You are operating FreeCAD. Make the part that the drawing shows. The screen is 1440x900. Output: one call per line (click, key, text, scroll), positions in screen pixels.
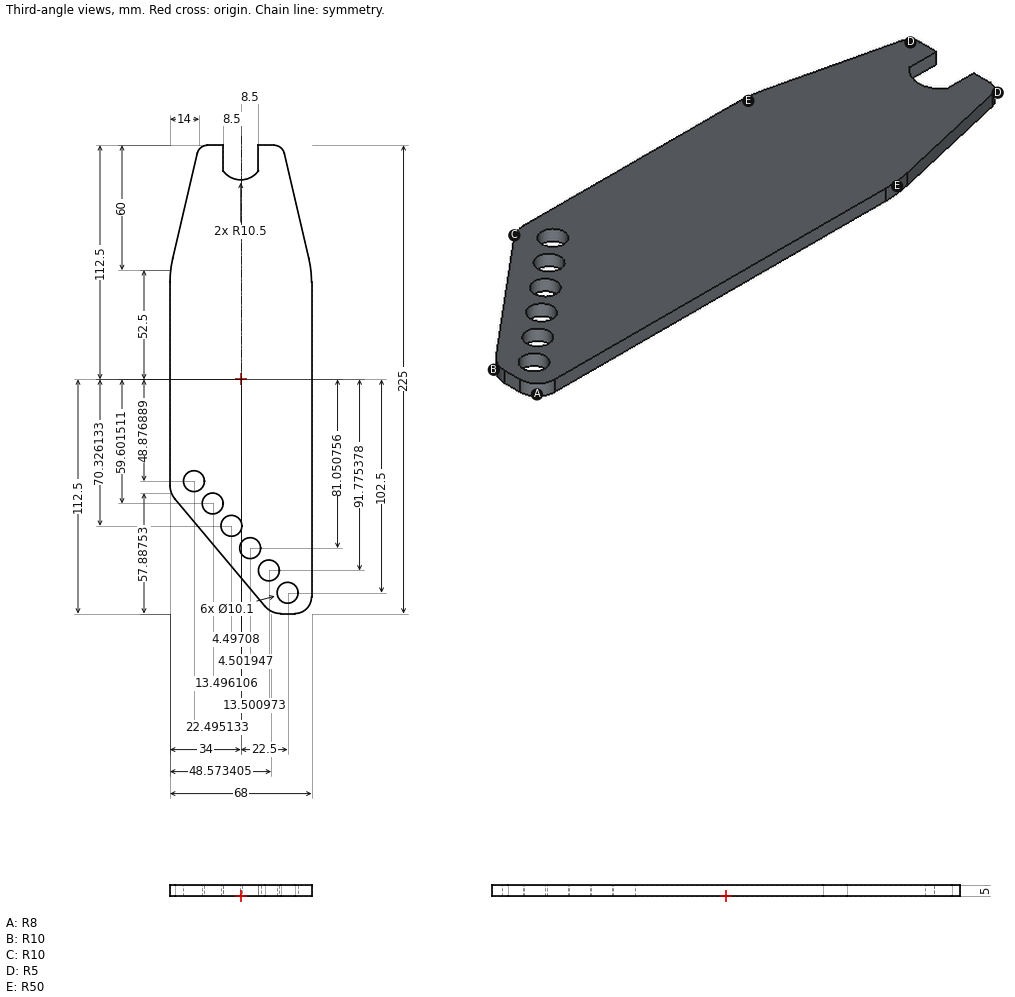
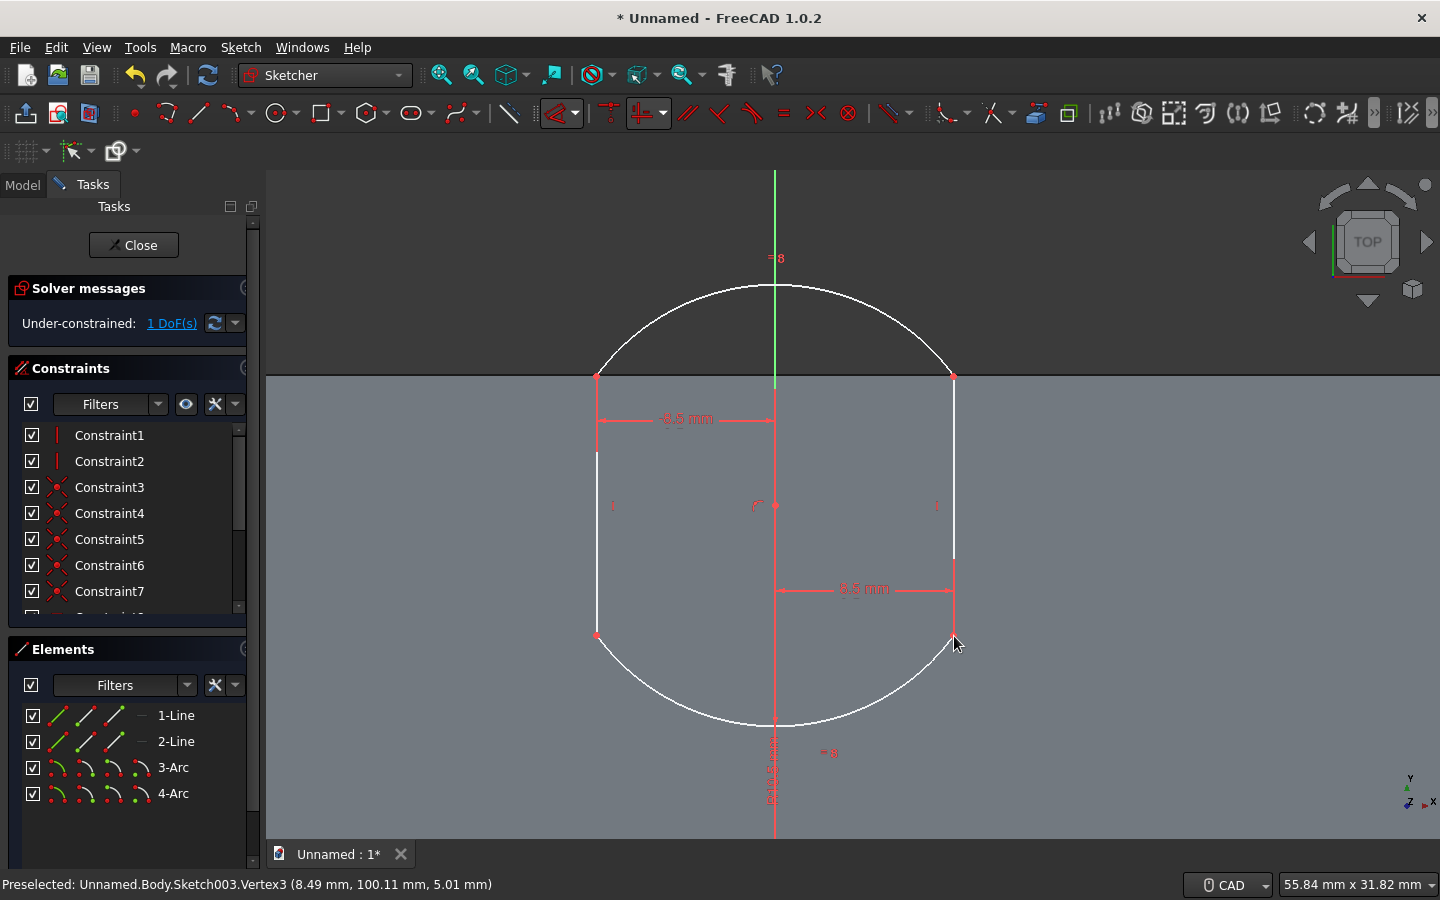
click(597, 376)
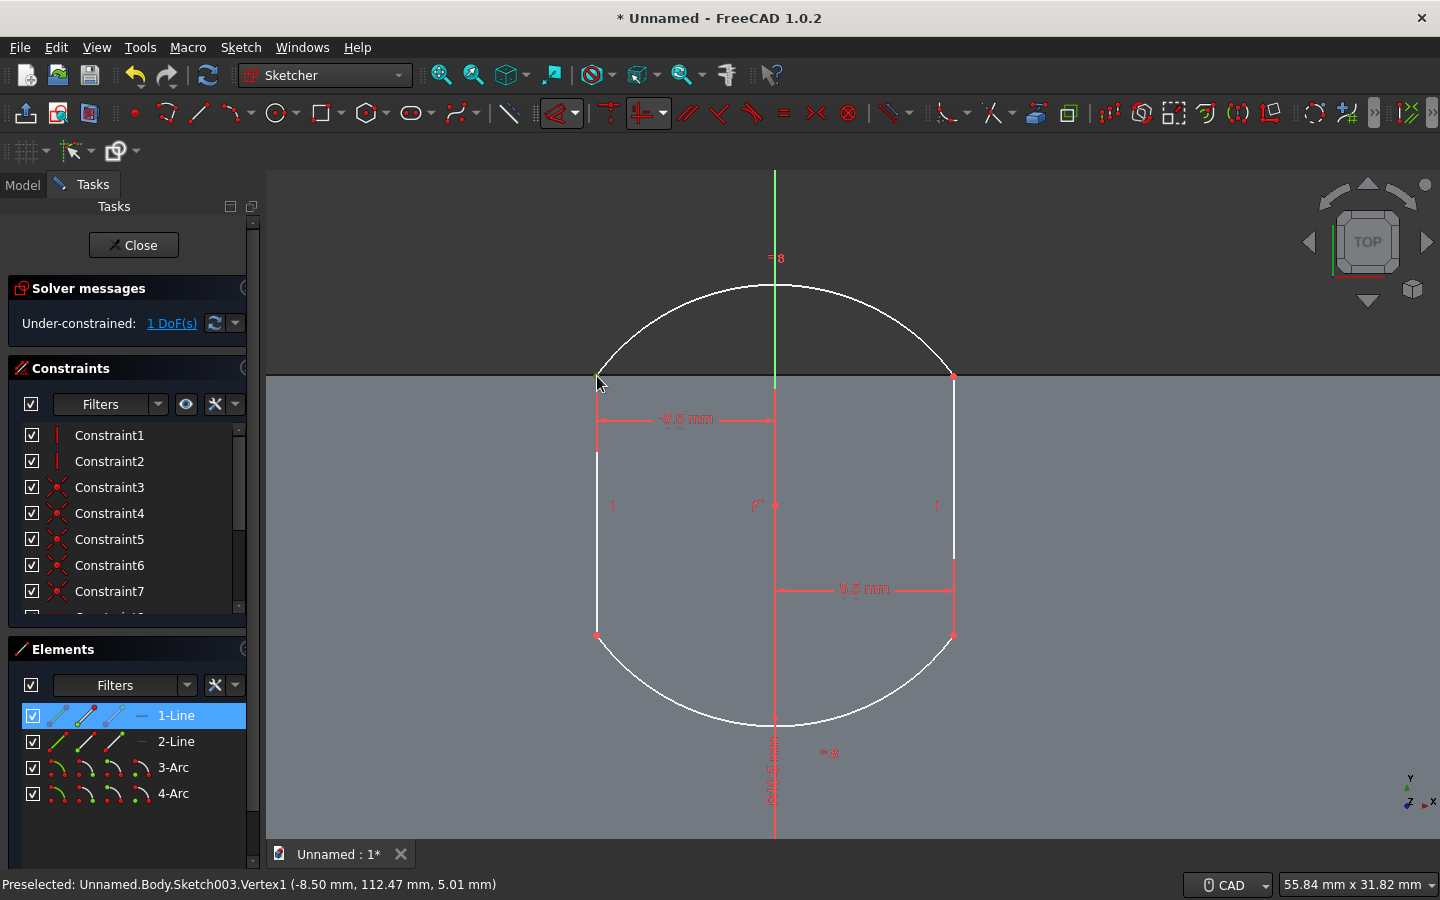
key(i)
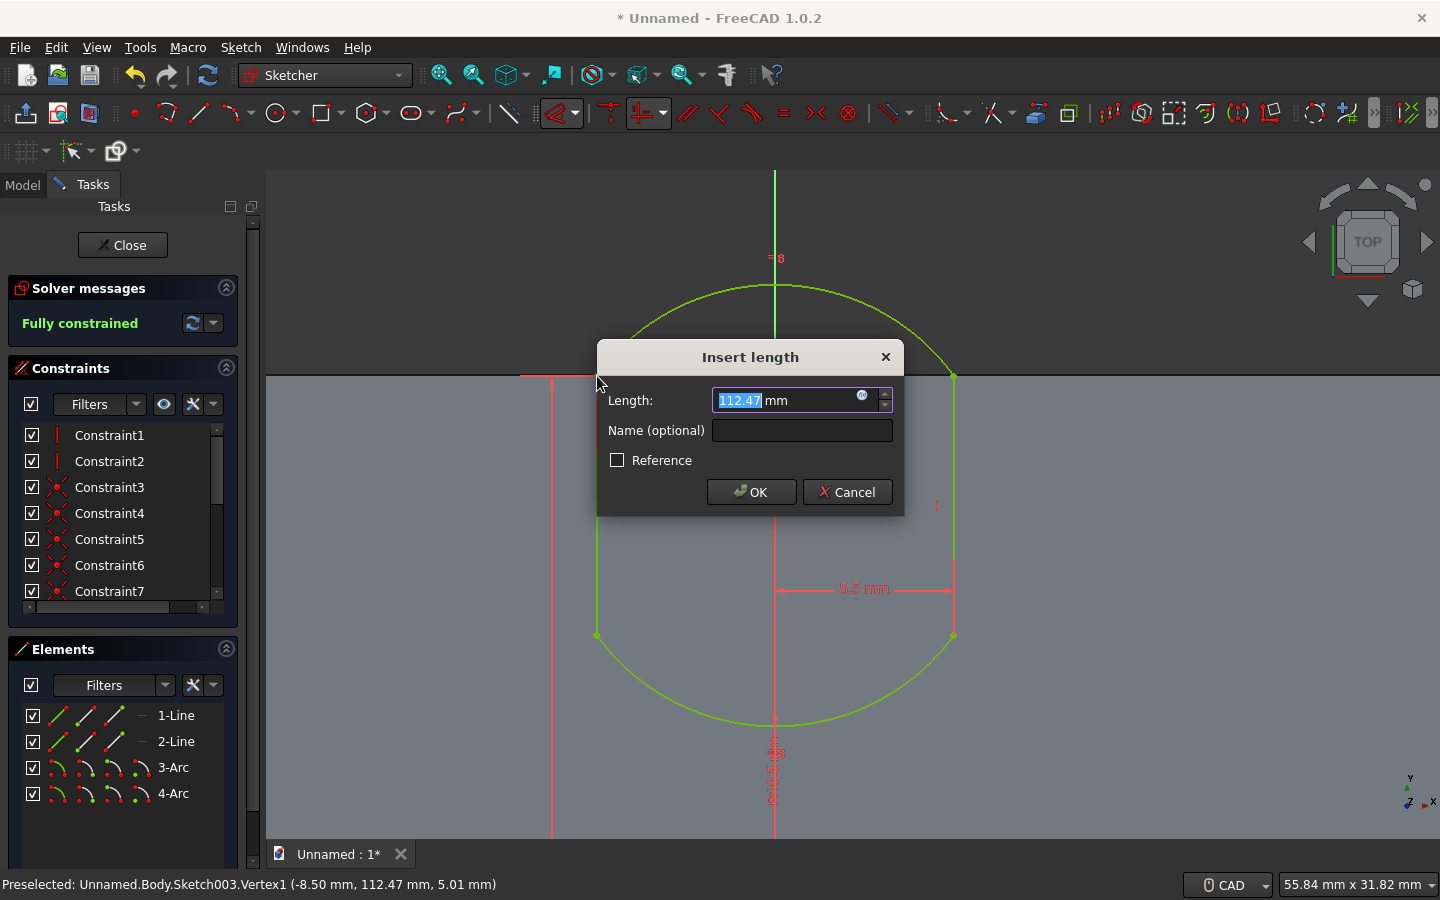
text(112.5)
key(Return)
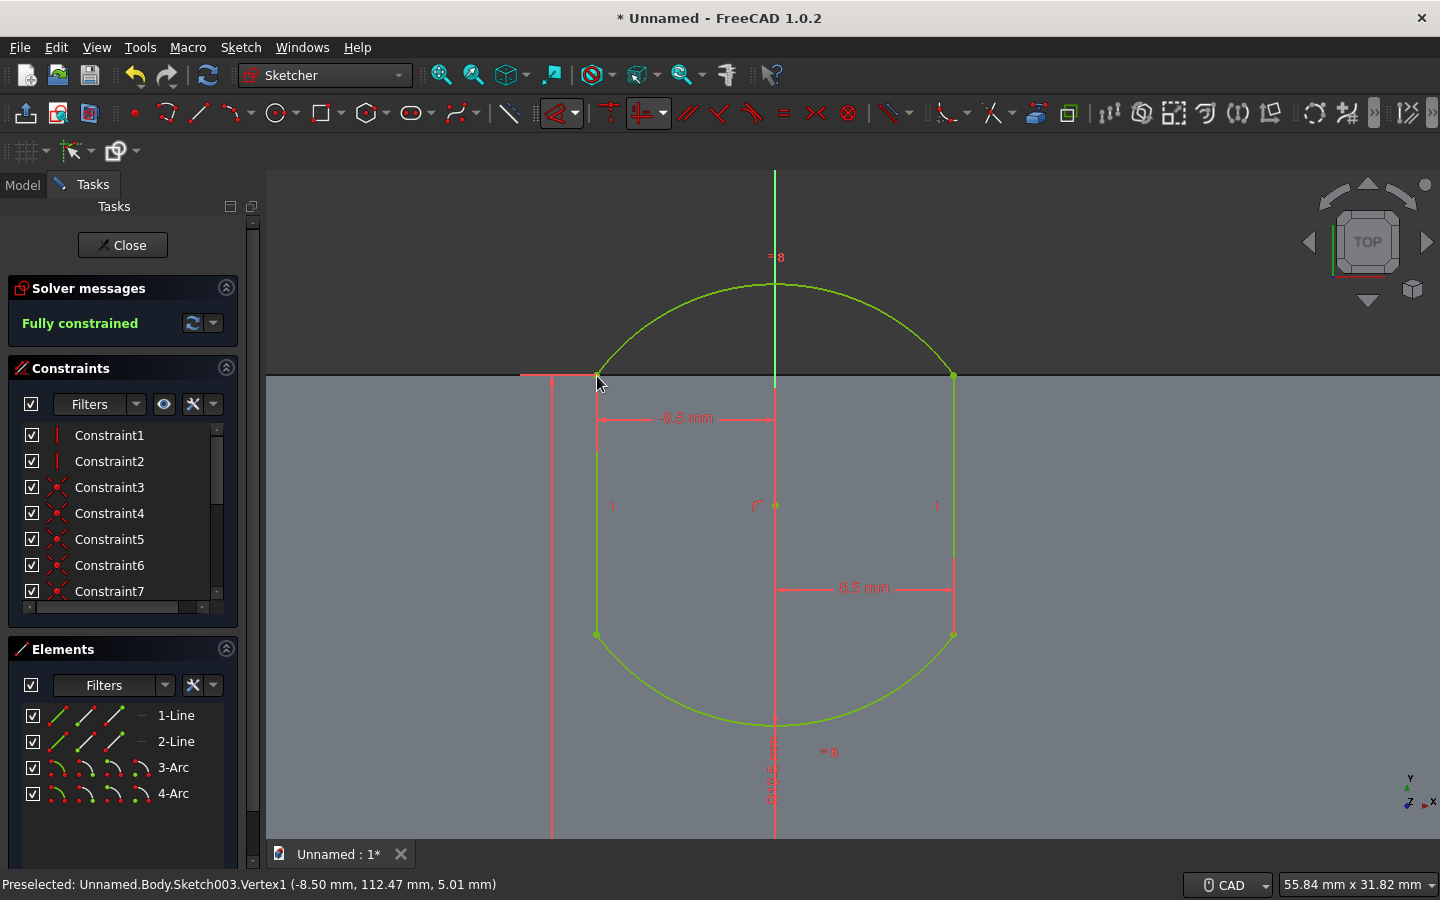
click(123, 245)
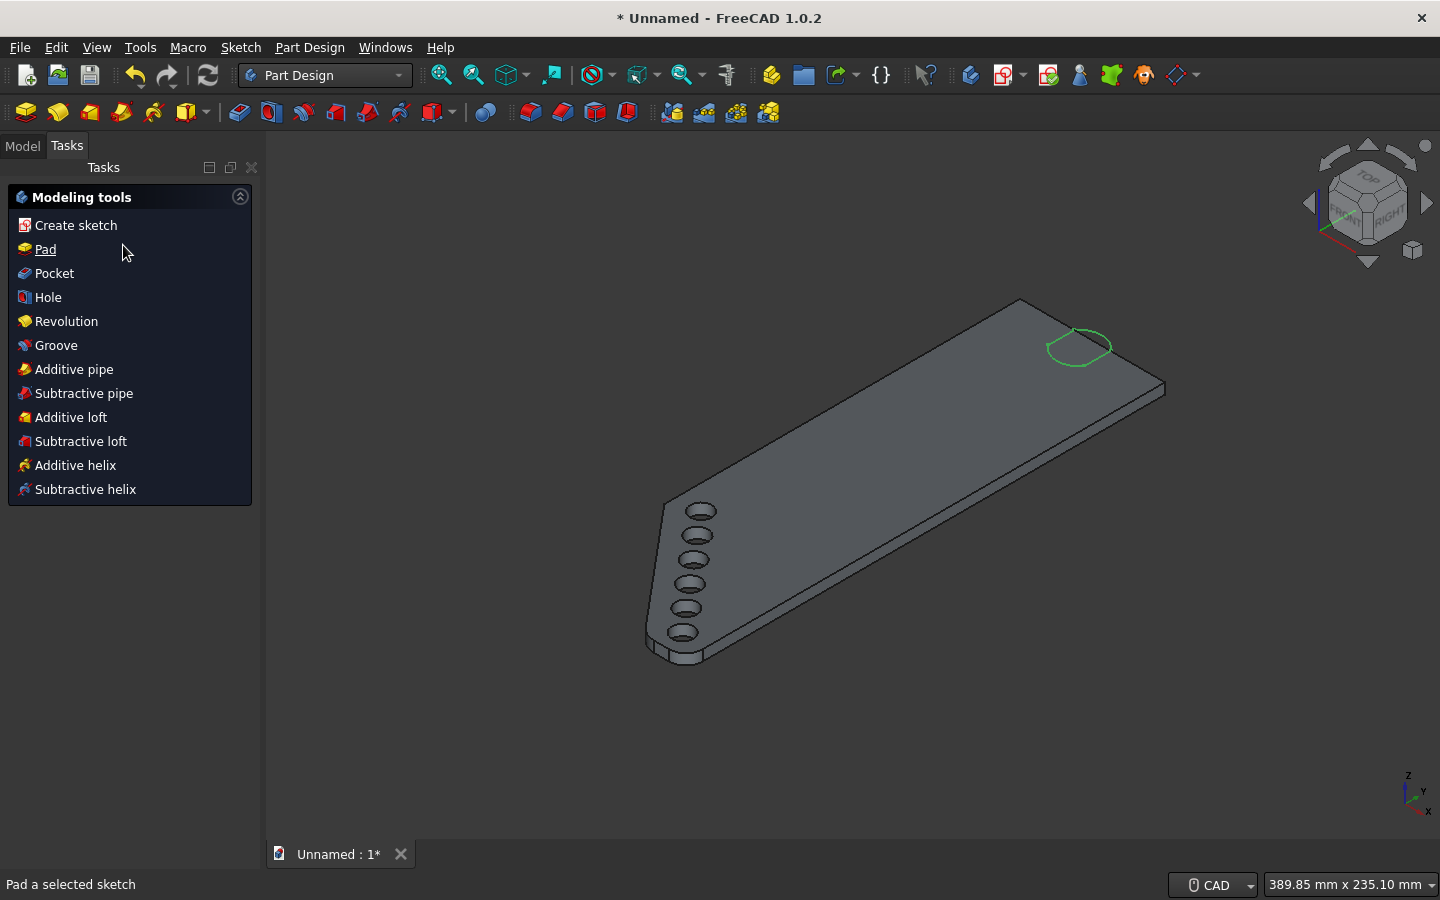
click(240, 112)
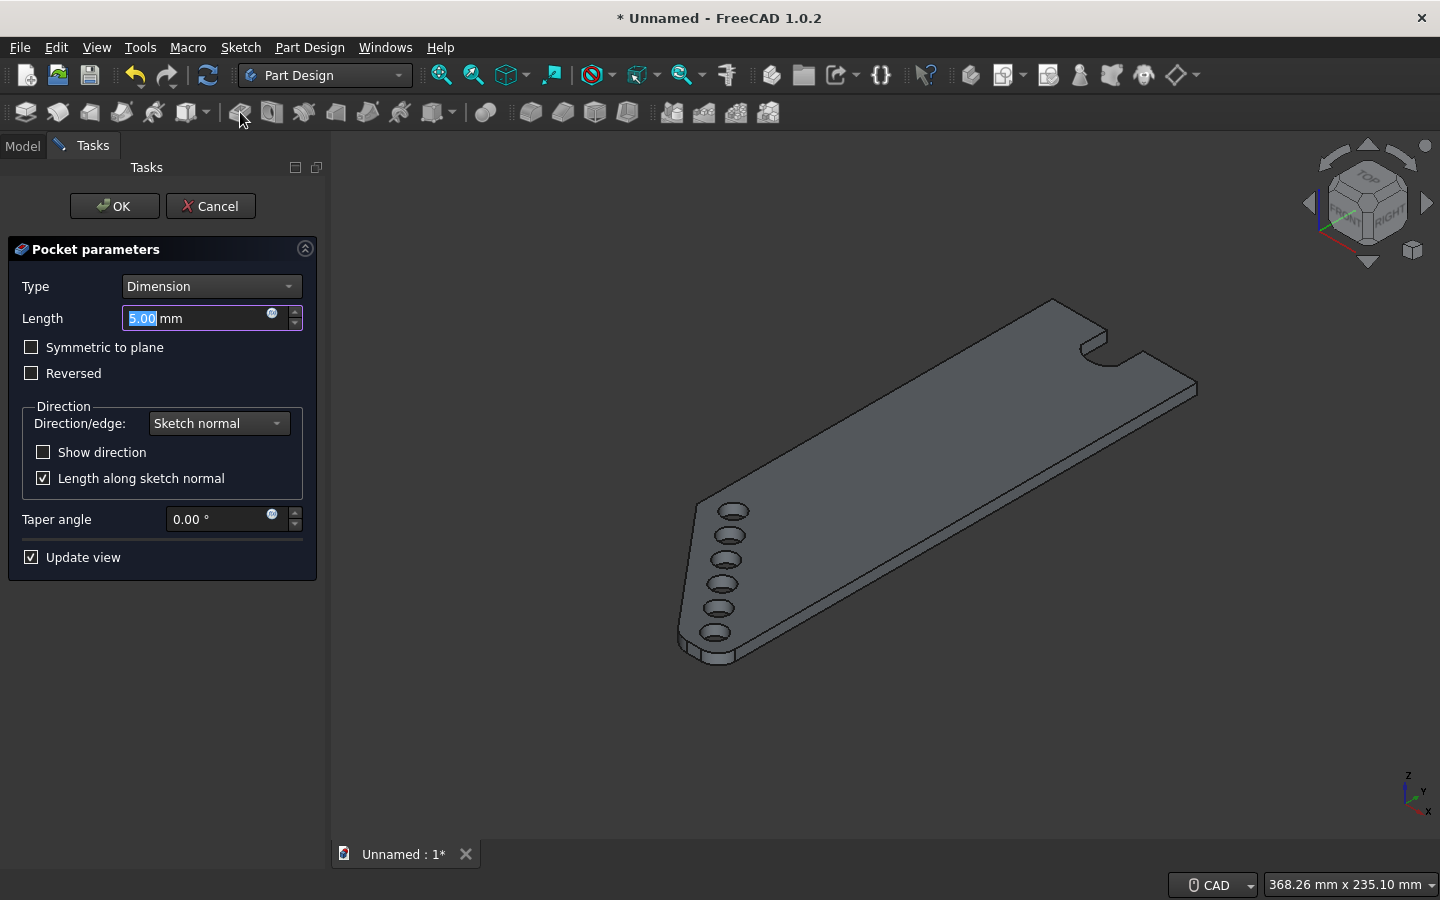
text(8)
key(Tab)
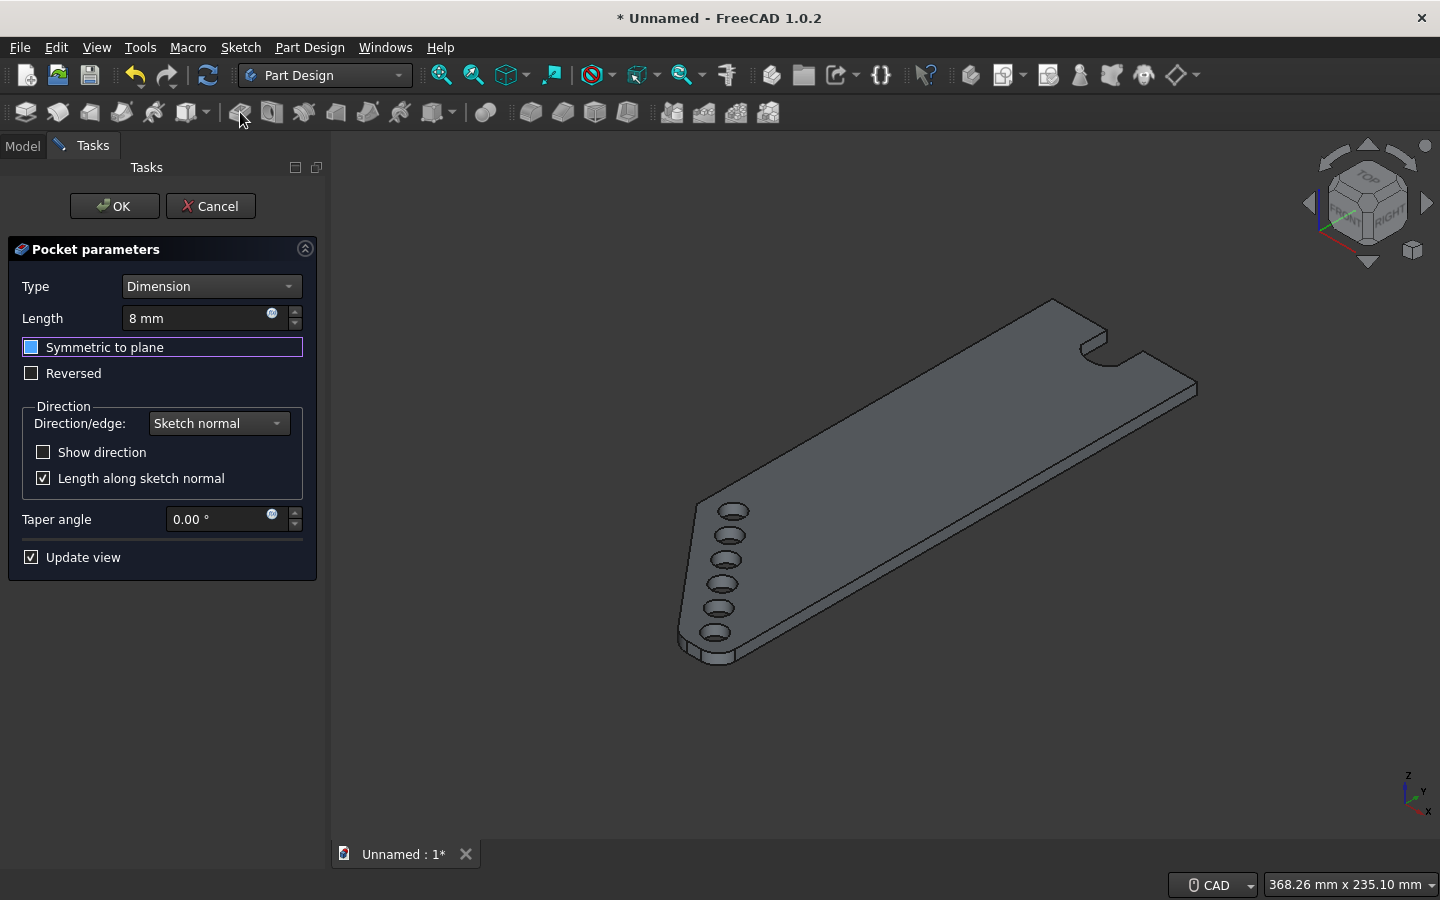
click(115, 206)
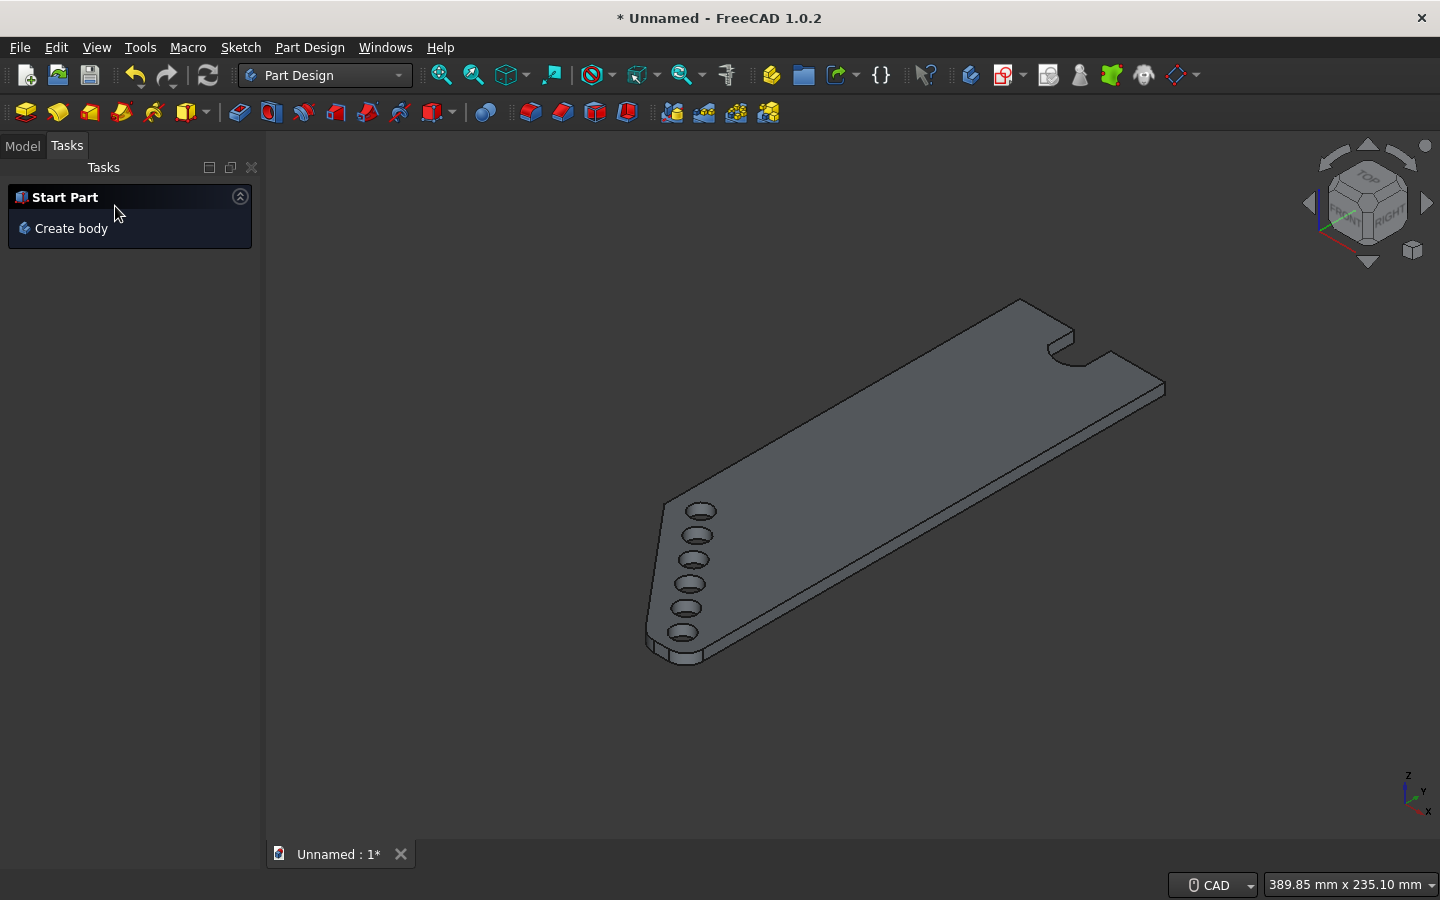
scroll(664, 509, up, 5)